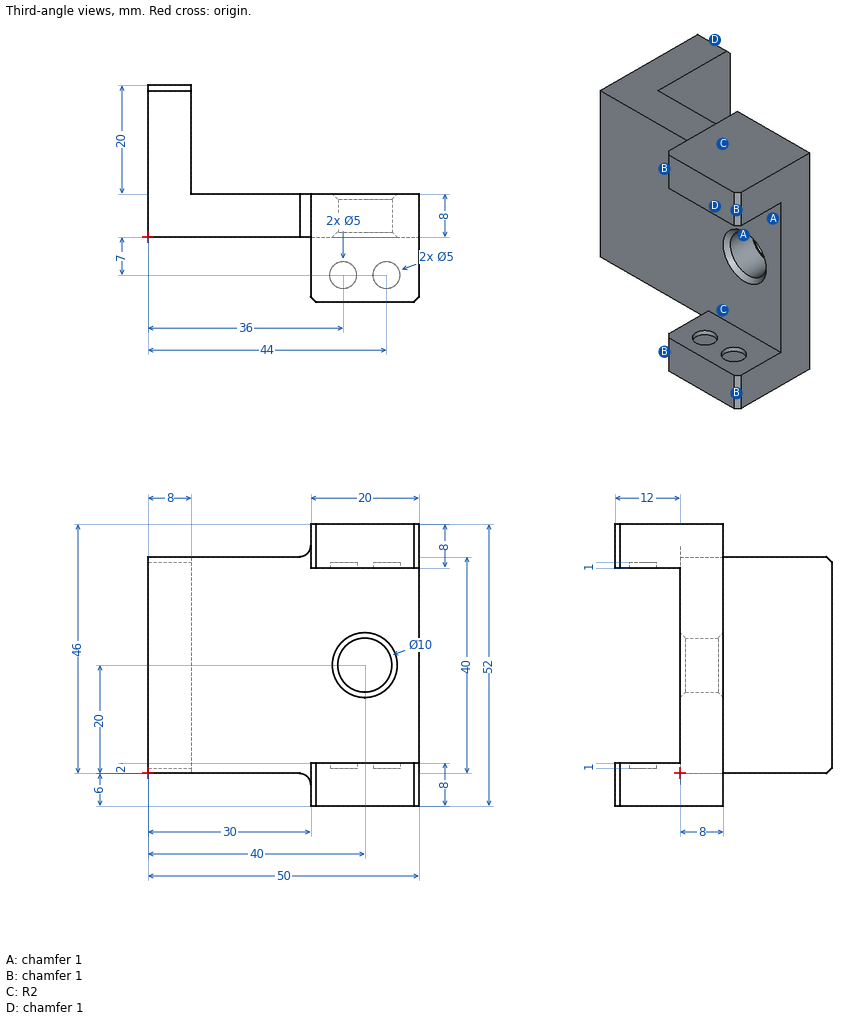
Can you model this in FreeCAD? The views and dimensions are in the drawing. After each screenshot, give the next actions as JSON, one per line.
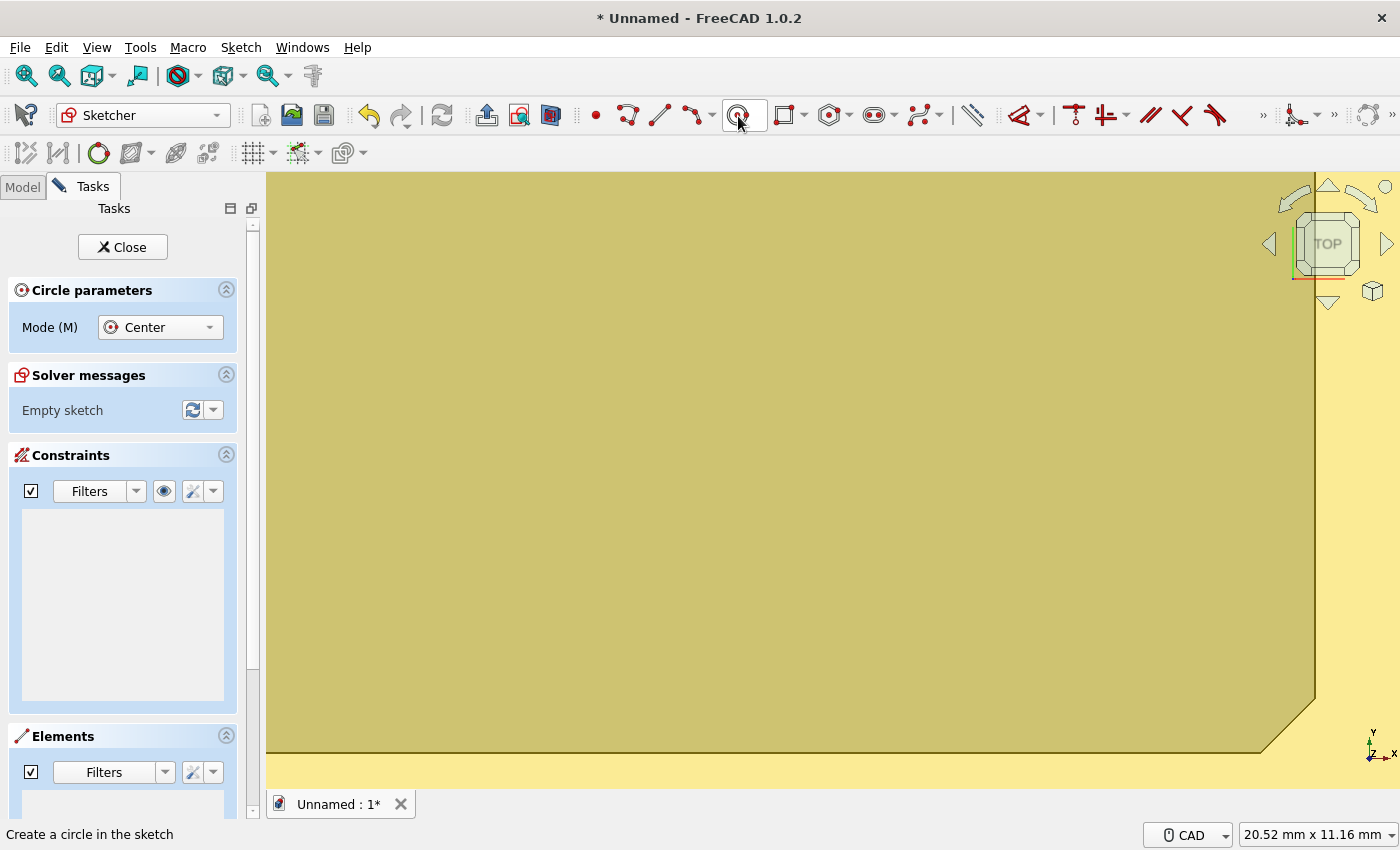
{"action": "left_click", "coordinate": [542, 477]}
{"action": "mouse_move", "coordinate": [639, 379]}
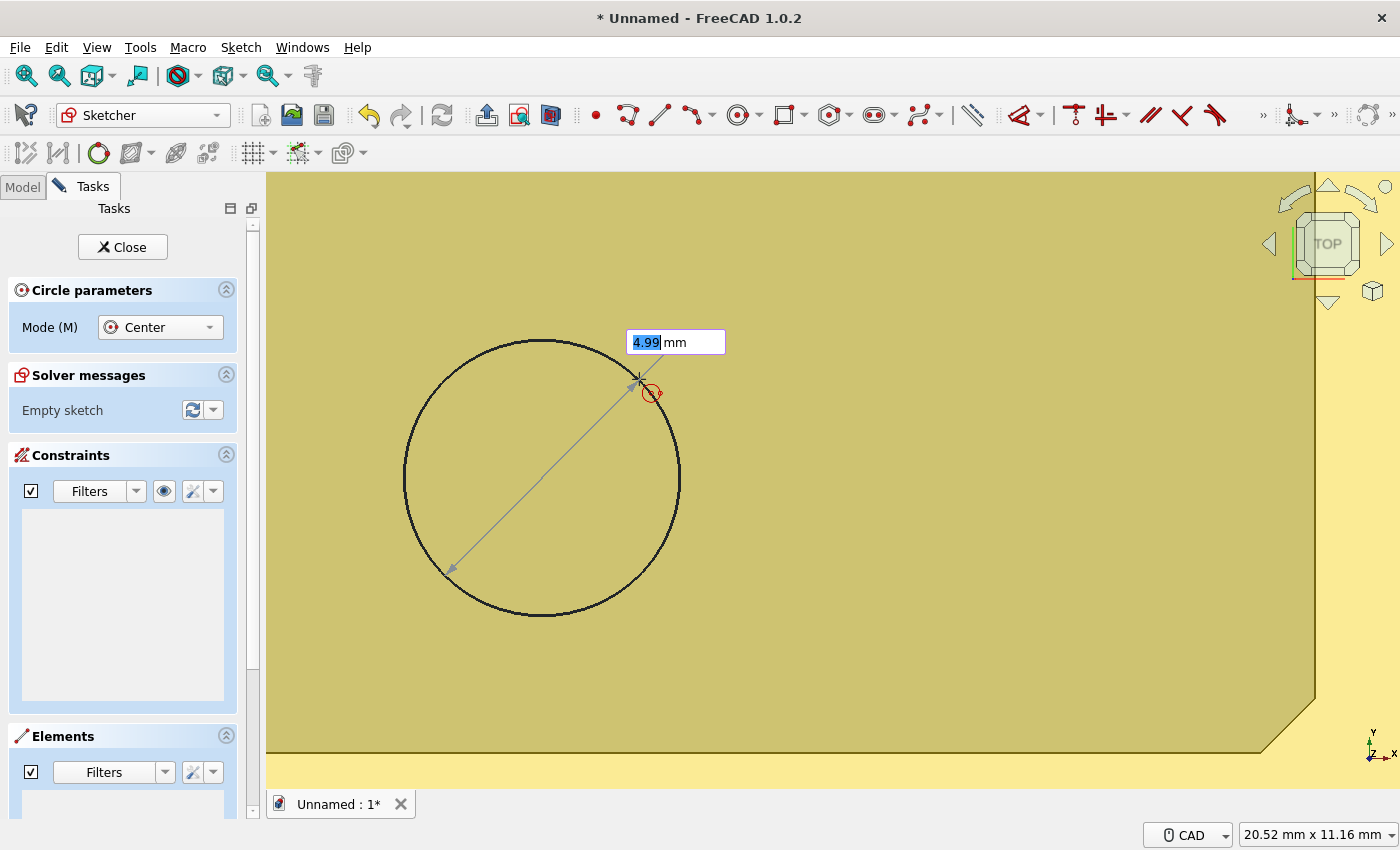
{"action": "type", "text": "5"}
{"action": "key", "text": "Return"}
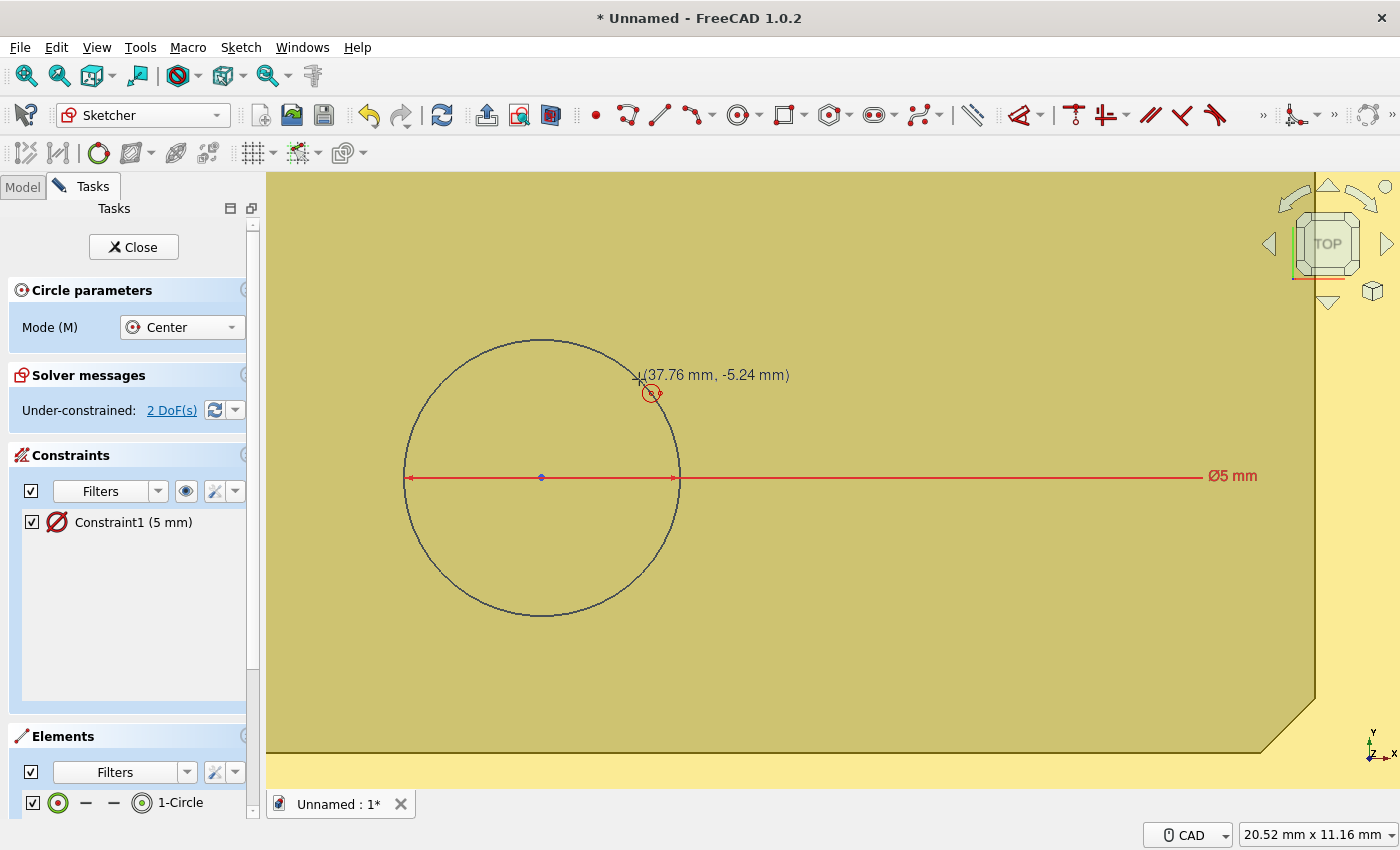
{"action": "left_click", "coordinate": [984, 477]}
{"action": "mouse_move", "coordinate": [1081, 379]}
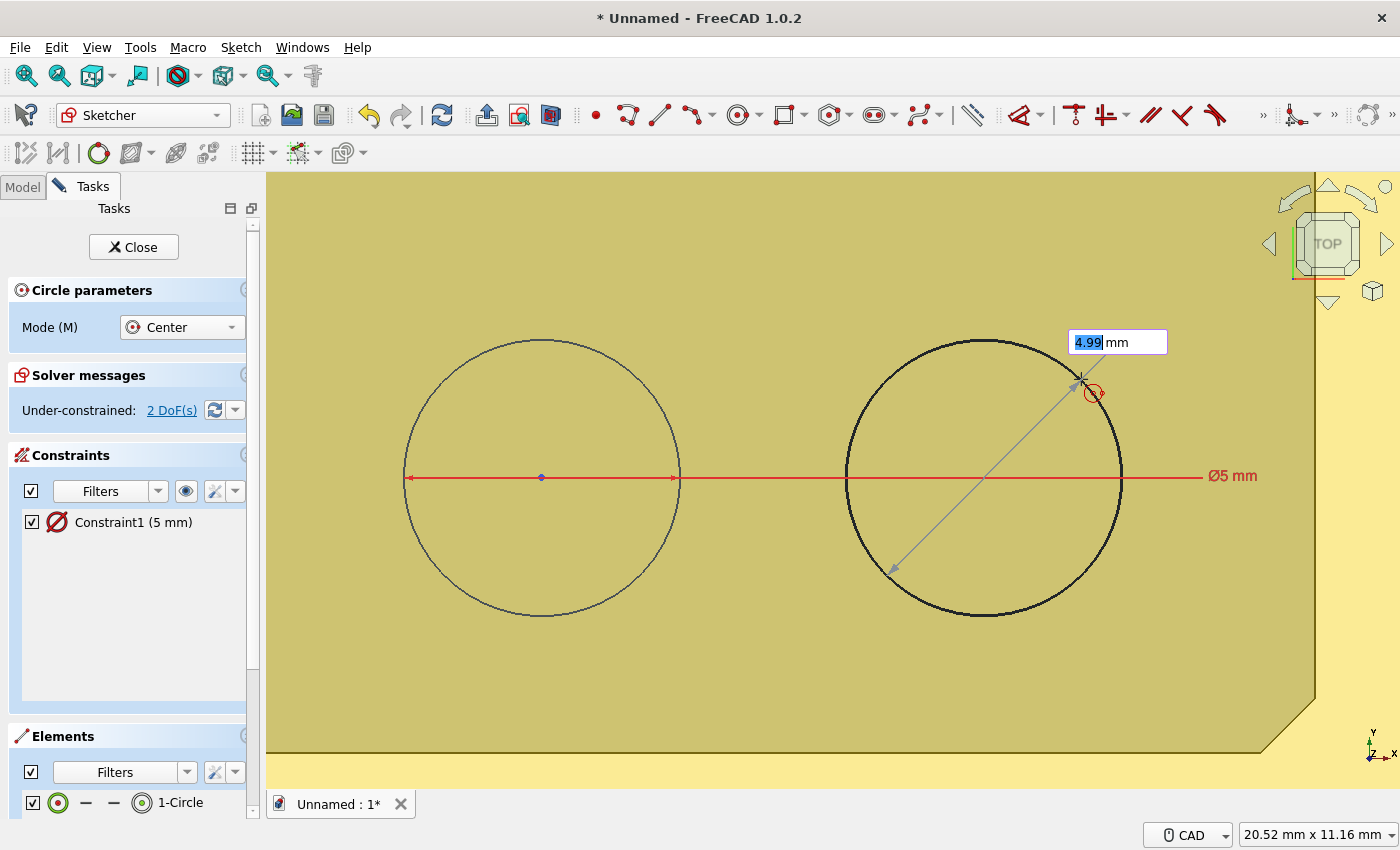
{"action": "type", "text": "5"}
{"action": "key", "text": "Return"}
{"action": "key", "text": "Escape"}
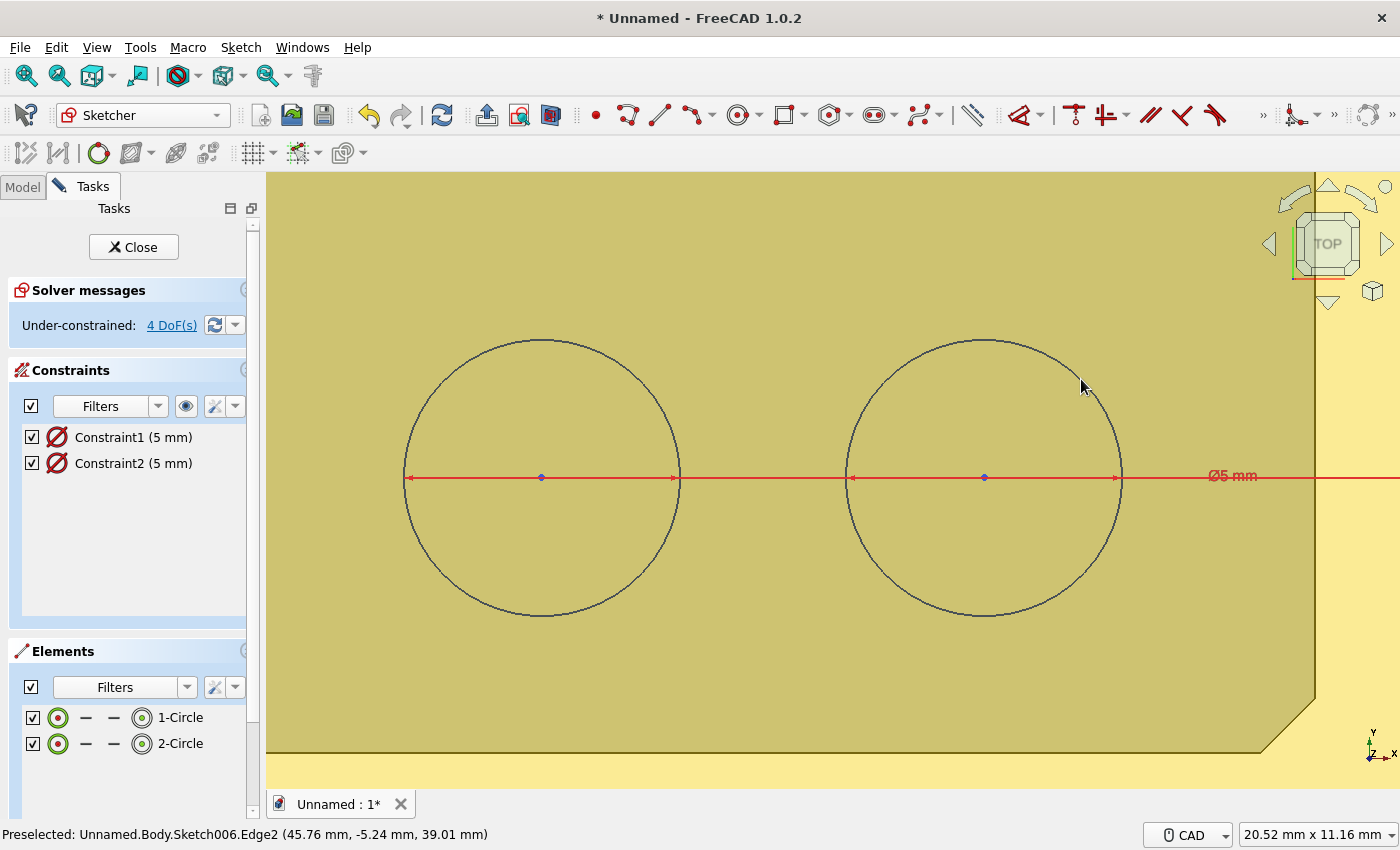
{"action": "left_click", "coordinate": [542, 478]}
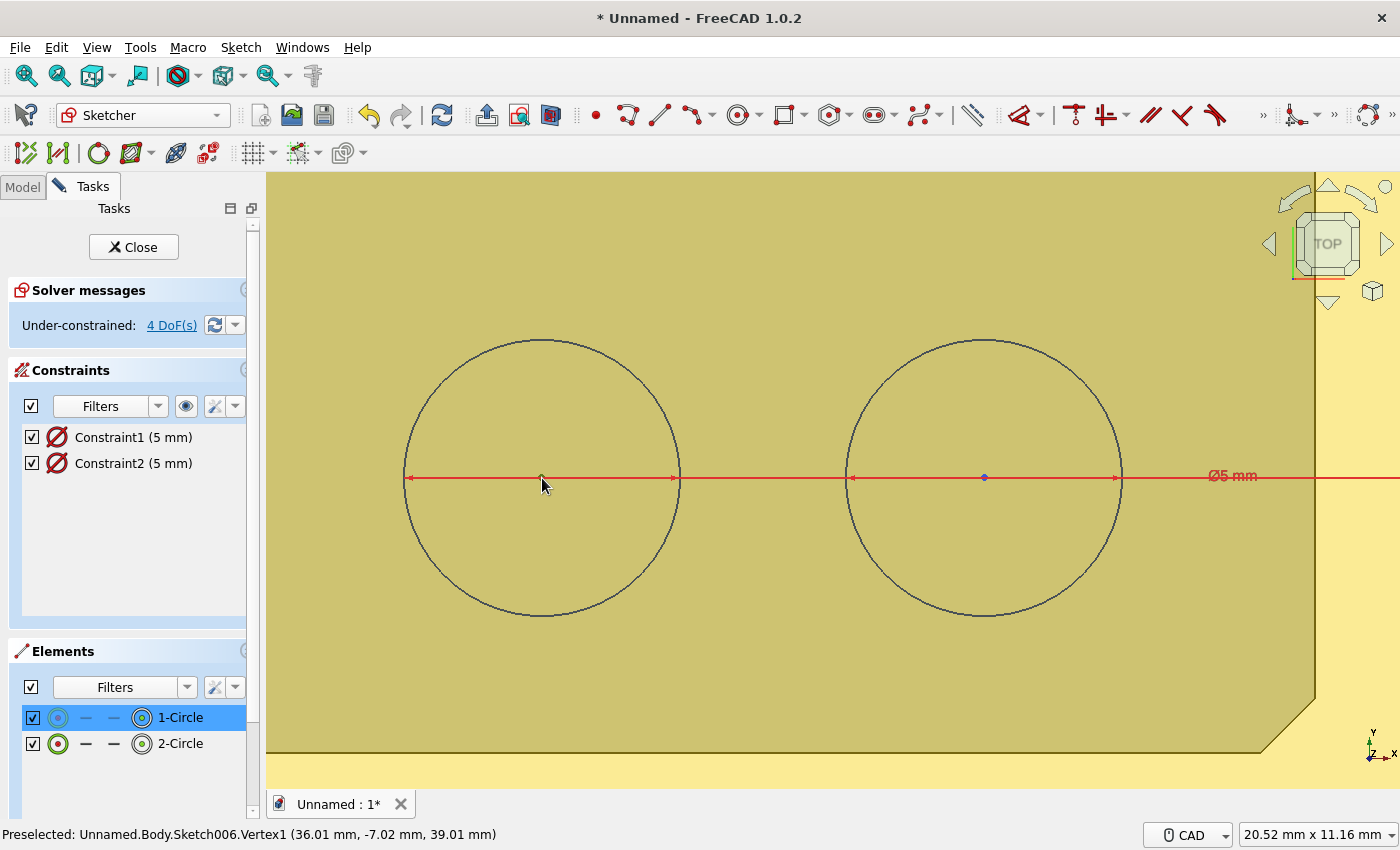
{"action": "left_click", "coordinate": [984, 478]}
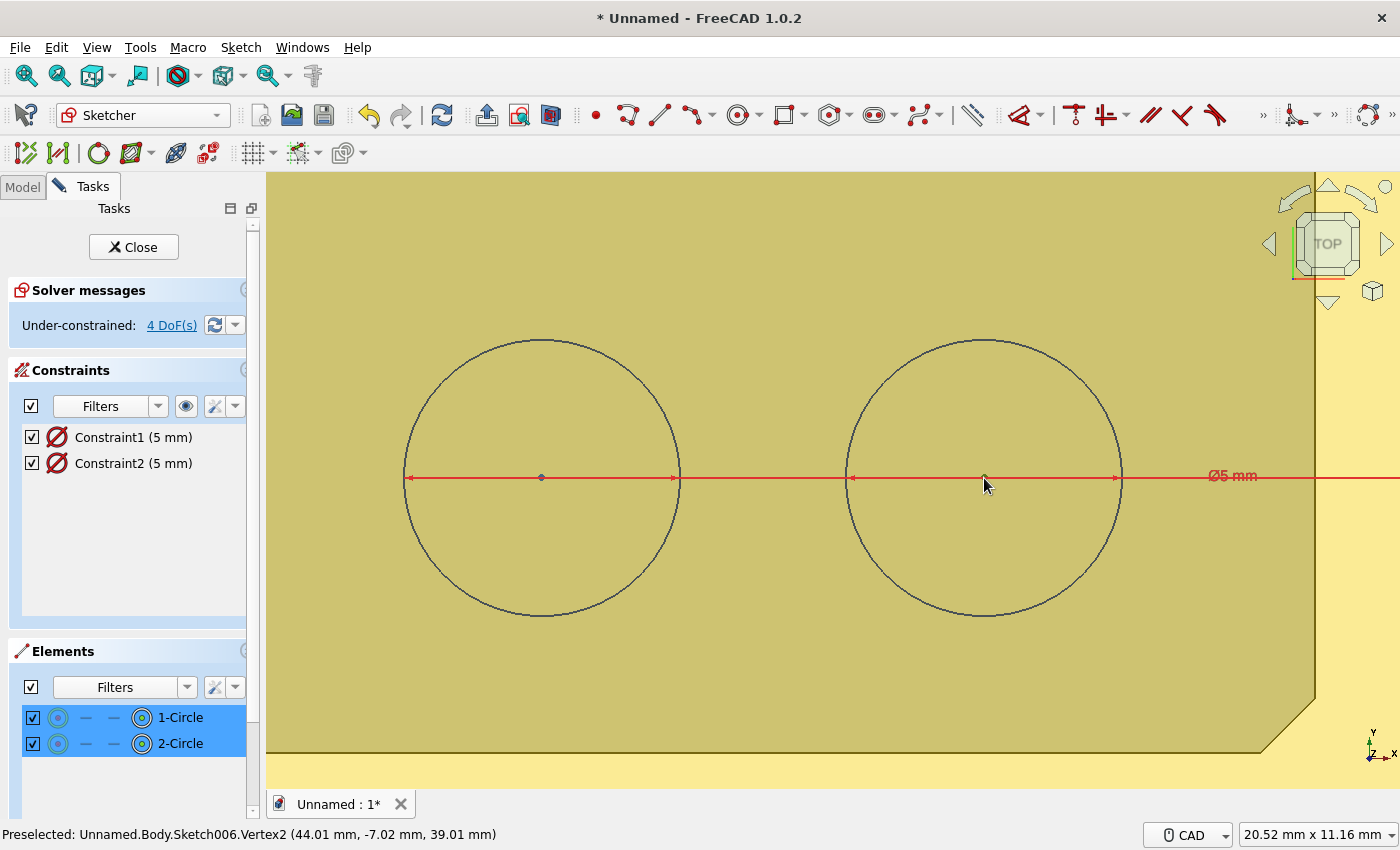
{"action": "left_click", "coordinate": [1128, 116]}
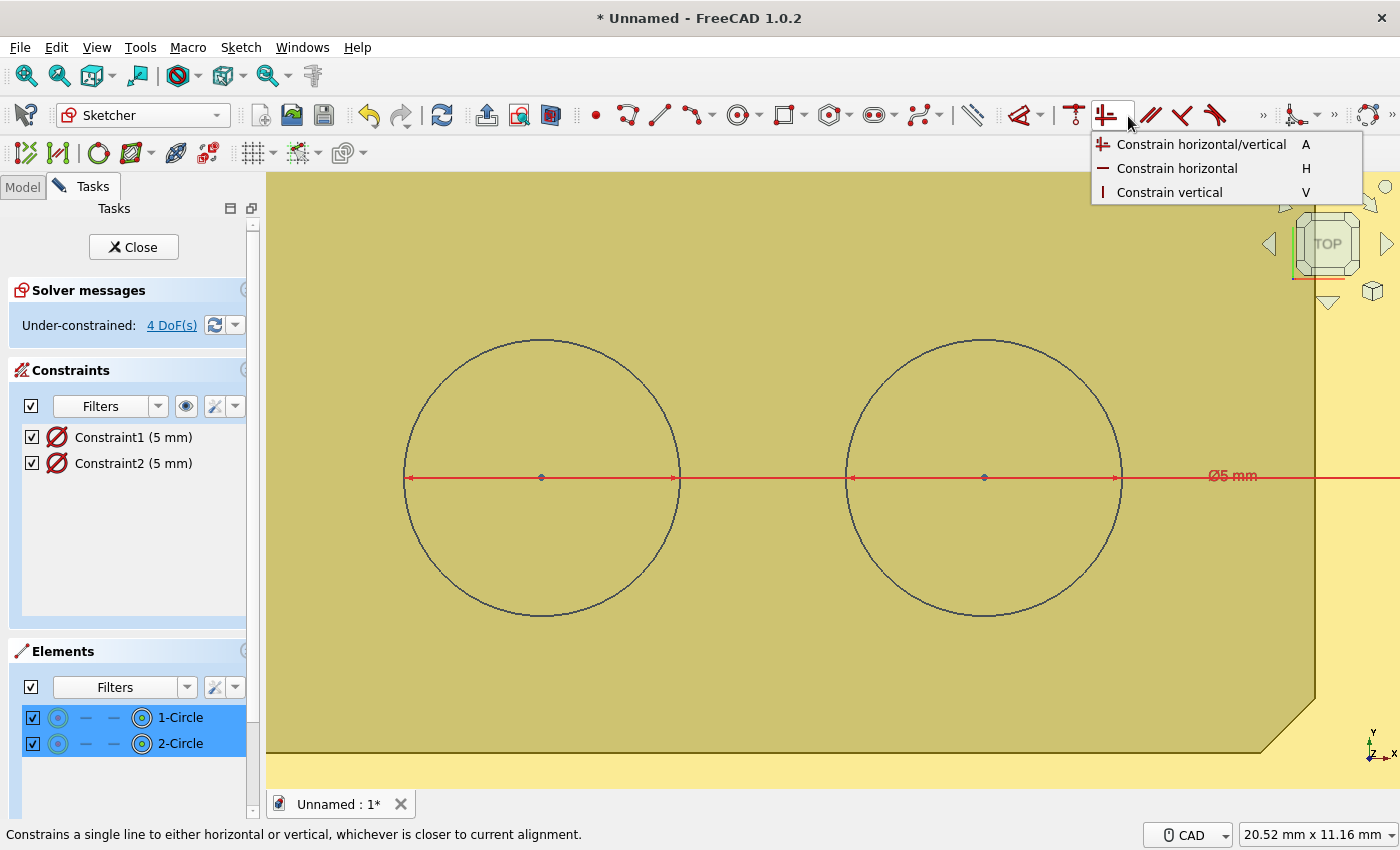
{"action": "left_click", "coordinate": [1227, 168]}